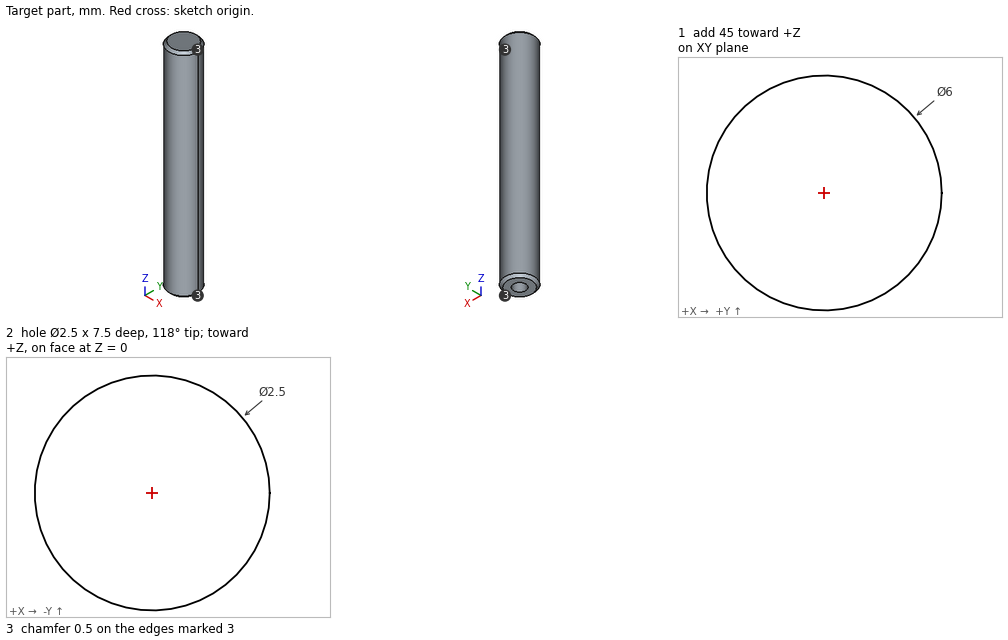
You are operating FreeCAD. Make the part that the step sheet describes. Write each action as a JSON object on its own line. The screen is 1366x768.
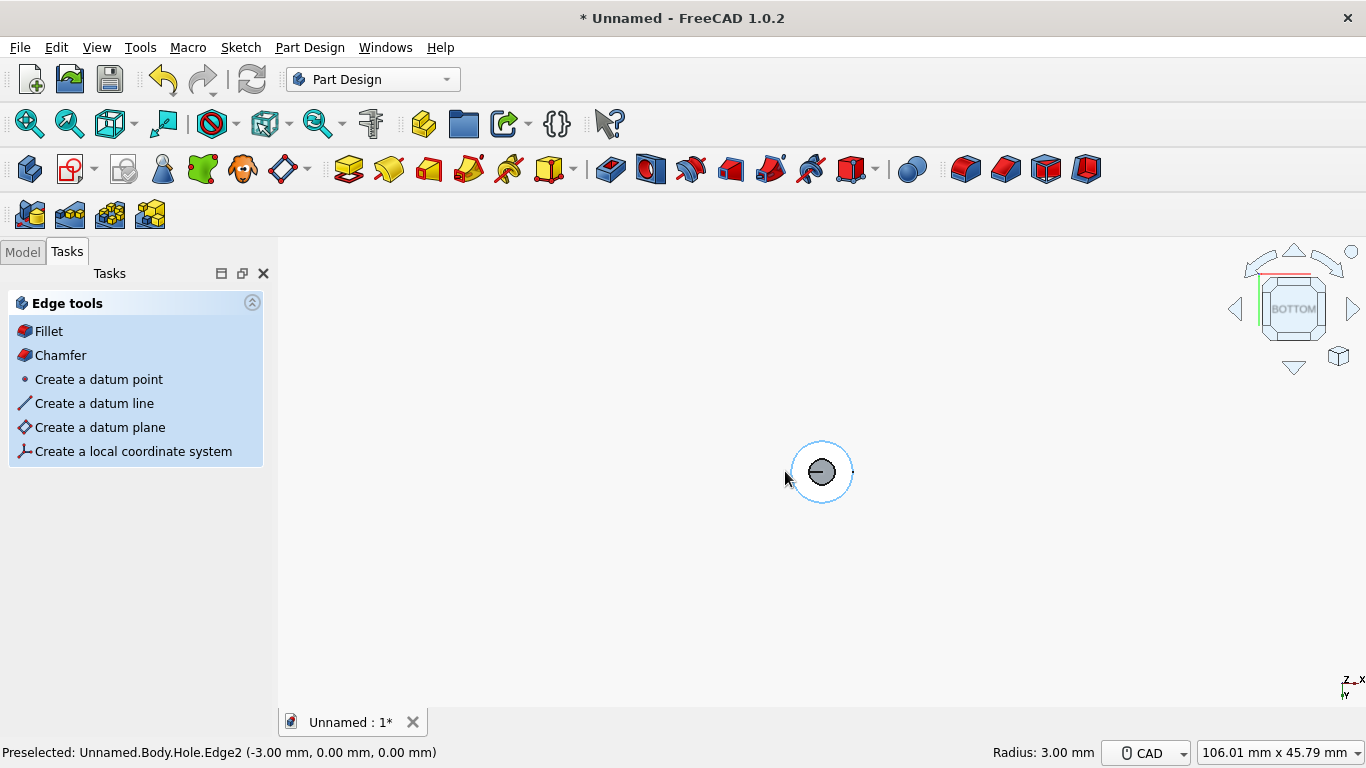
{"action": "key", "text": "0"}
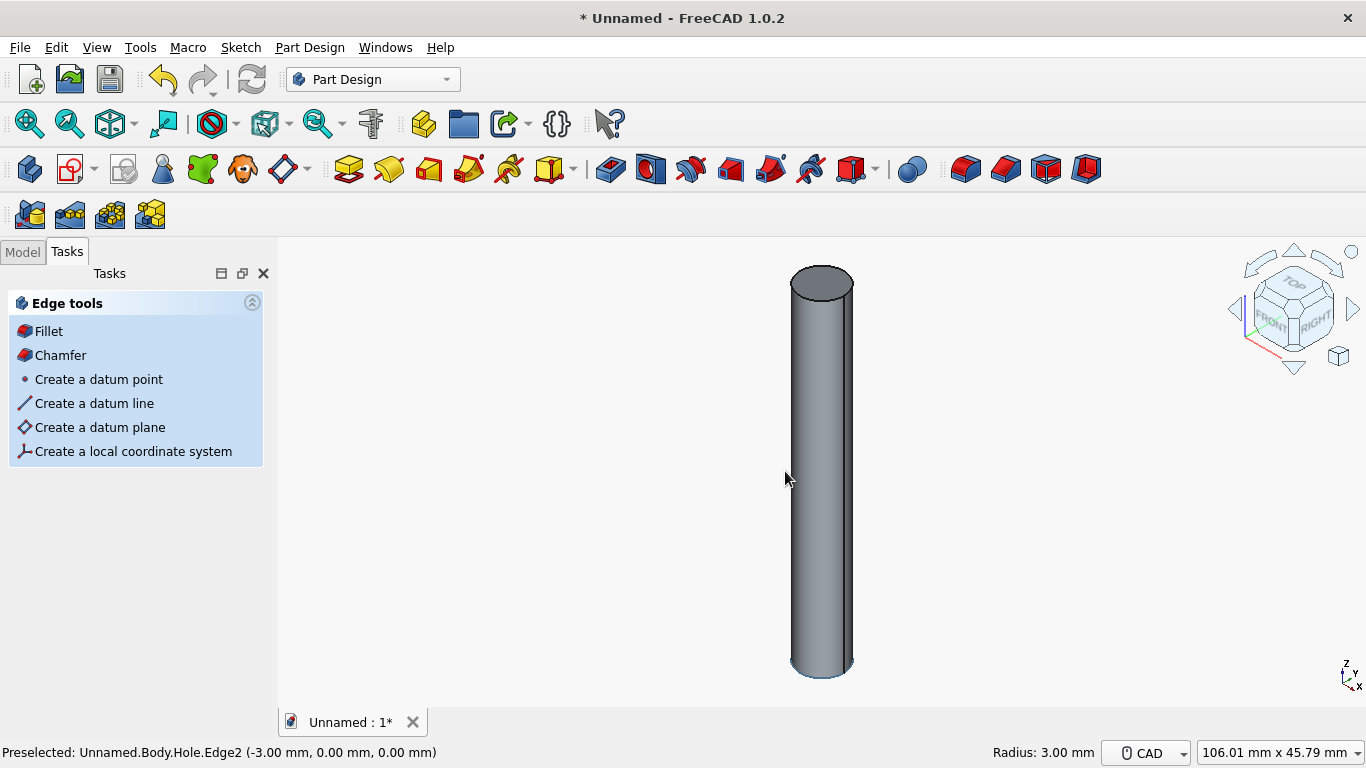
{"action": "left_click", "coordinate": [795, 291], "text": "ctrl"}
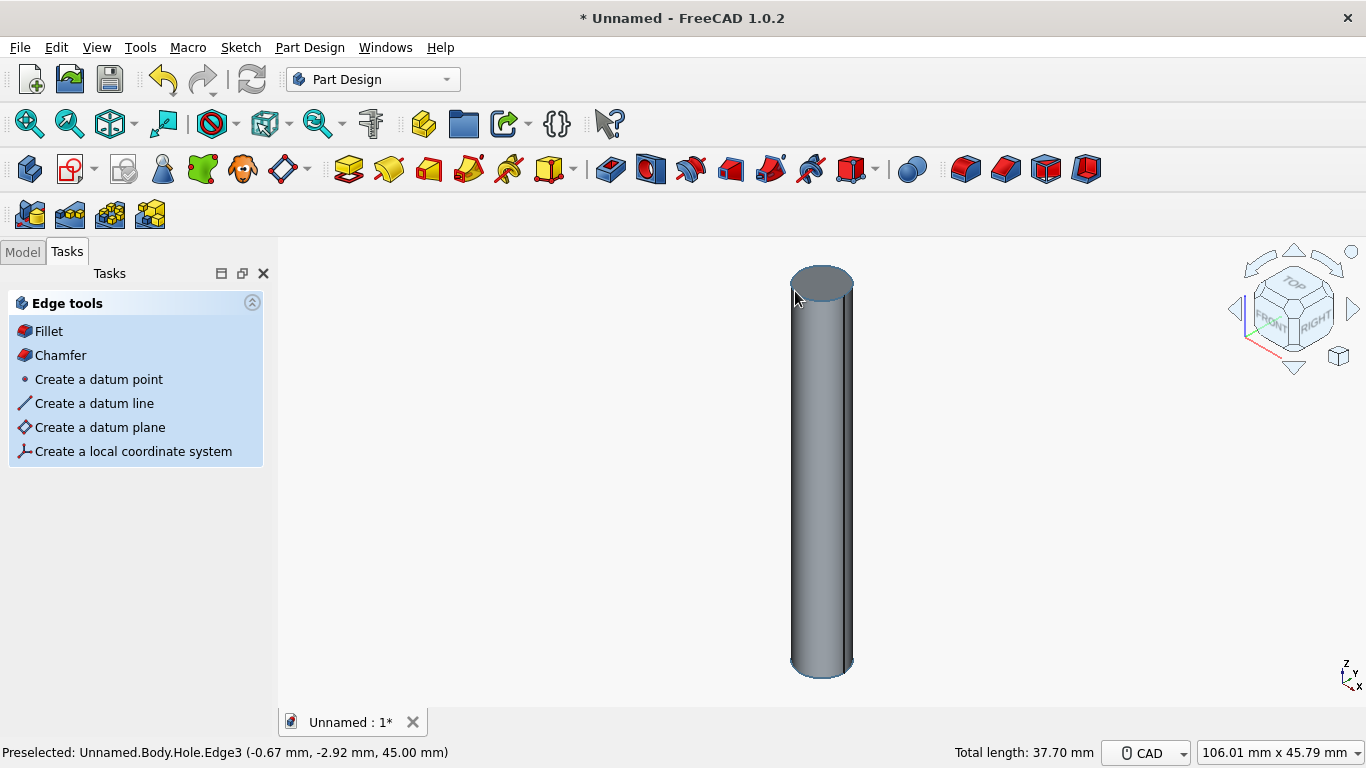
{"action": "left_click", "coordinate": [1006, 170]}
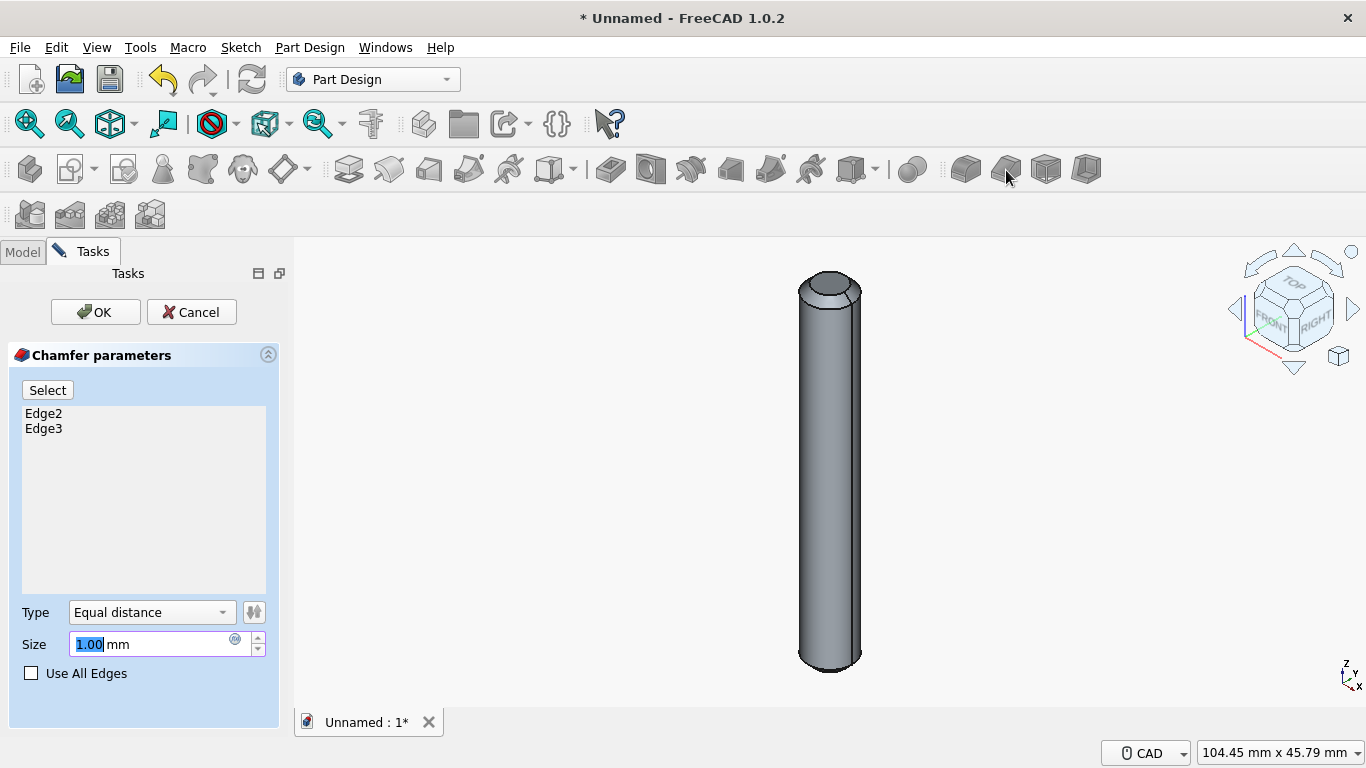
{"action": "type", "text": "0.5"}
{"action": "key", "text": "Tab"}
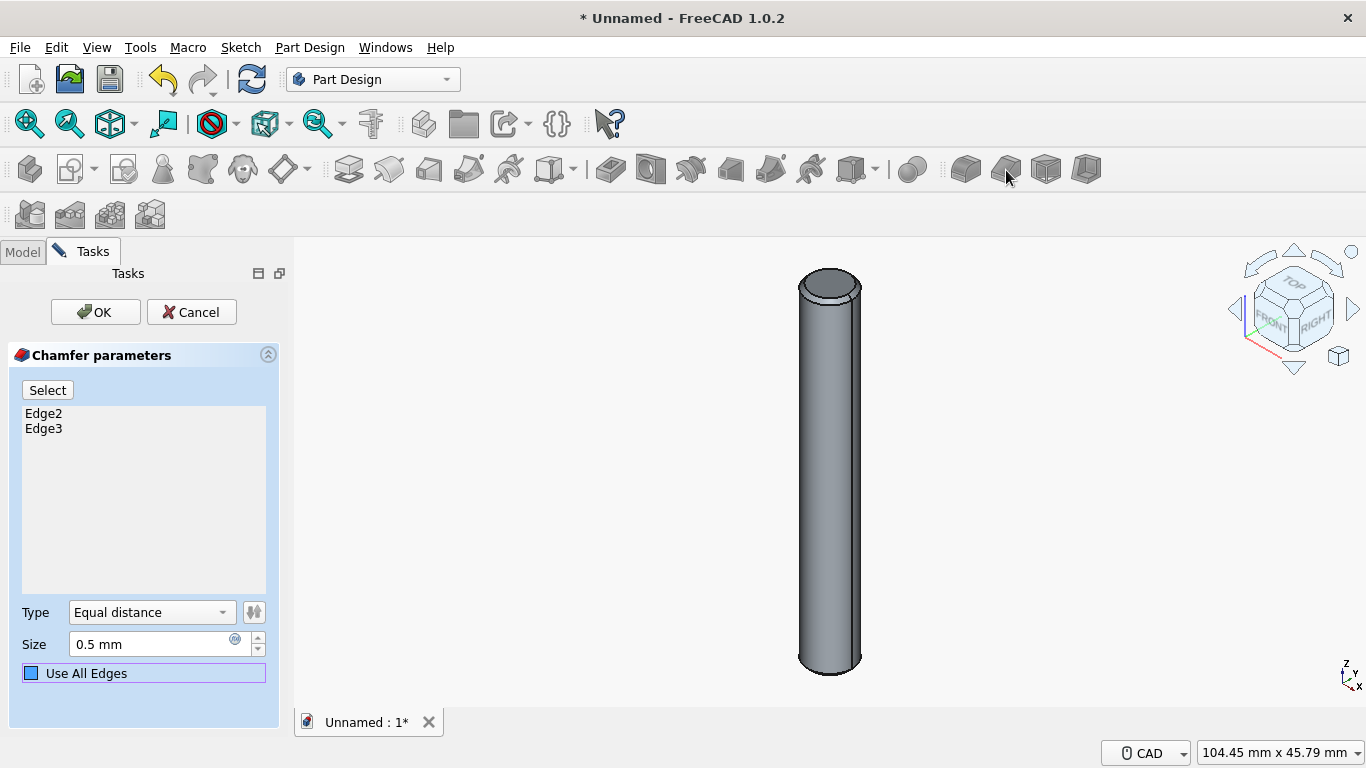
{"action": "left_click", "coordinate": [96, 312]}